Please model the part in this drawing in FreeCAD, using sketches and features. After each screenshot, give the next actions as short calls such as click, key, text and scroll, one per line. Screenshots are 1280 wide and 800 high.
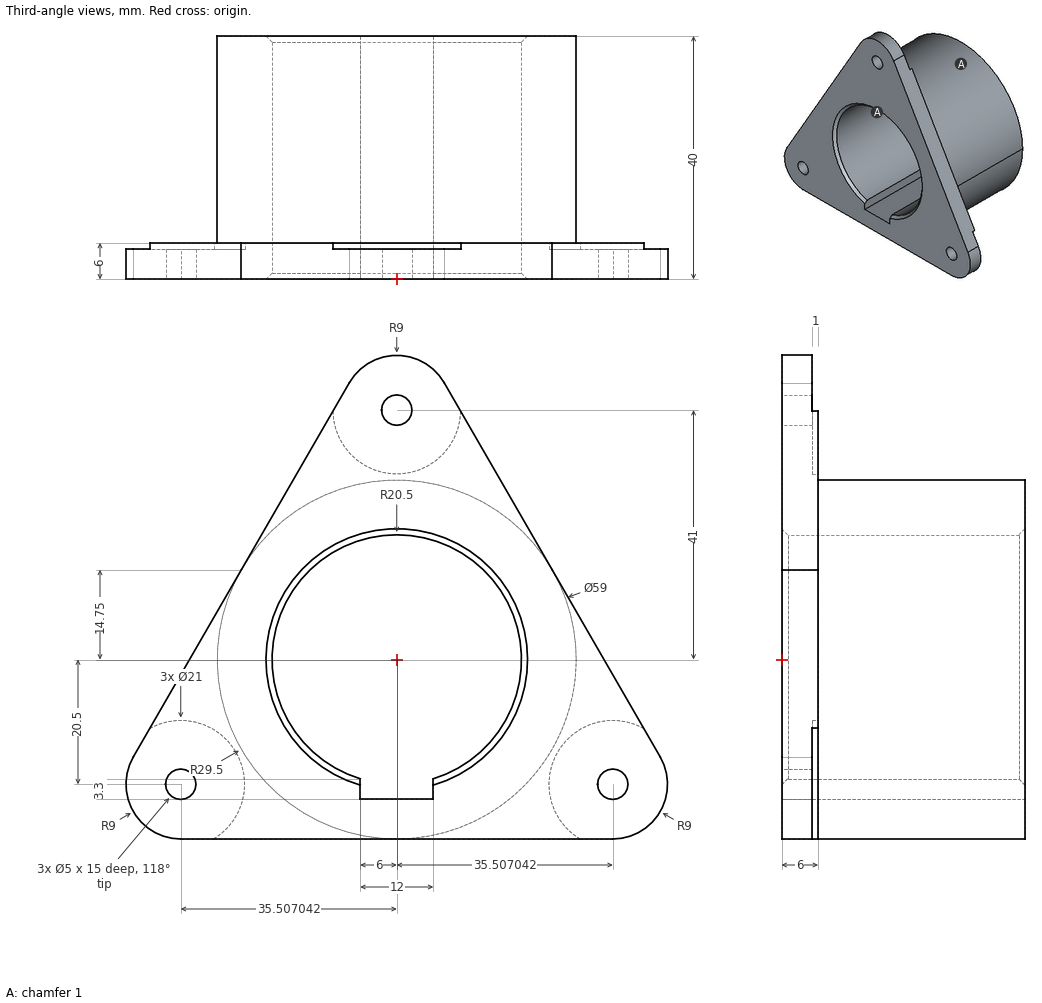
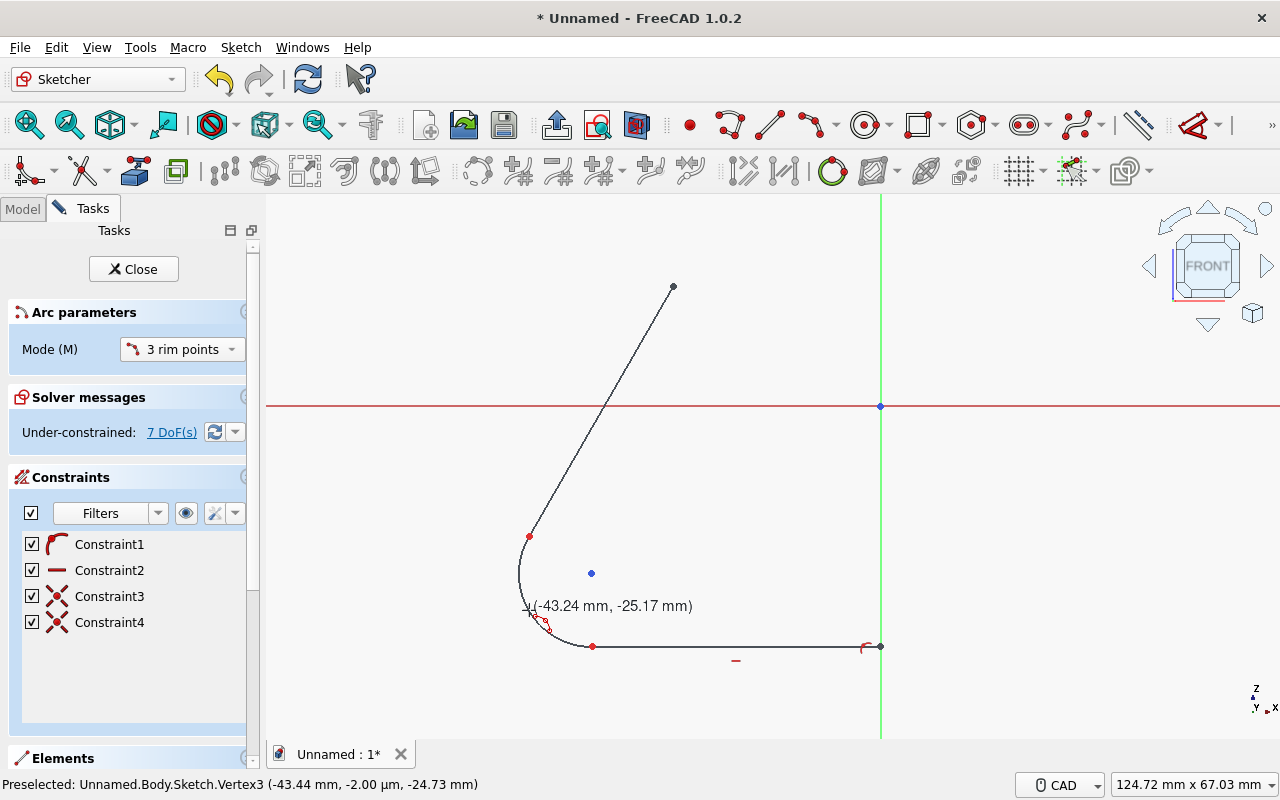
click(673, 287)
click(881, 647)
click(673, 526)
key(Escape)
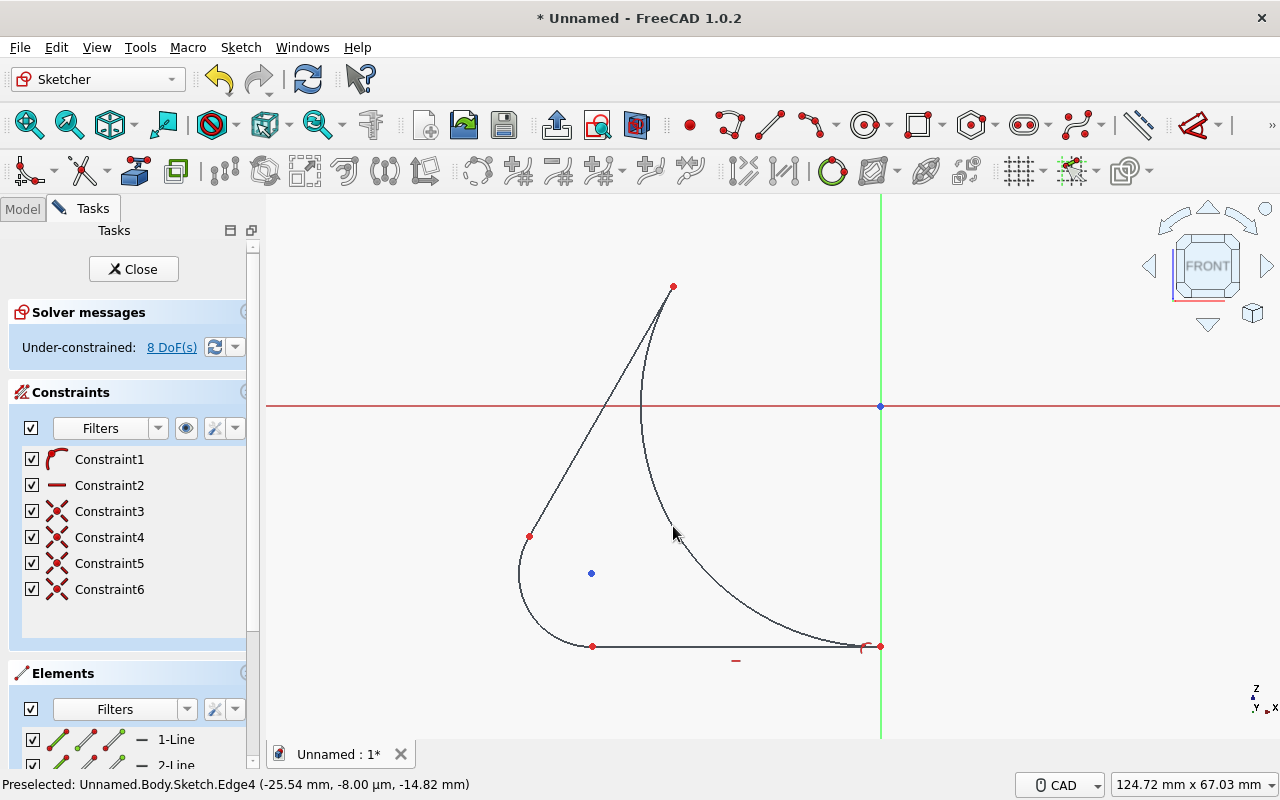
click(794, 647)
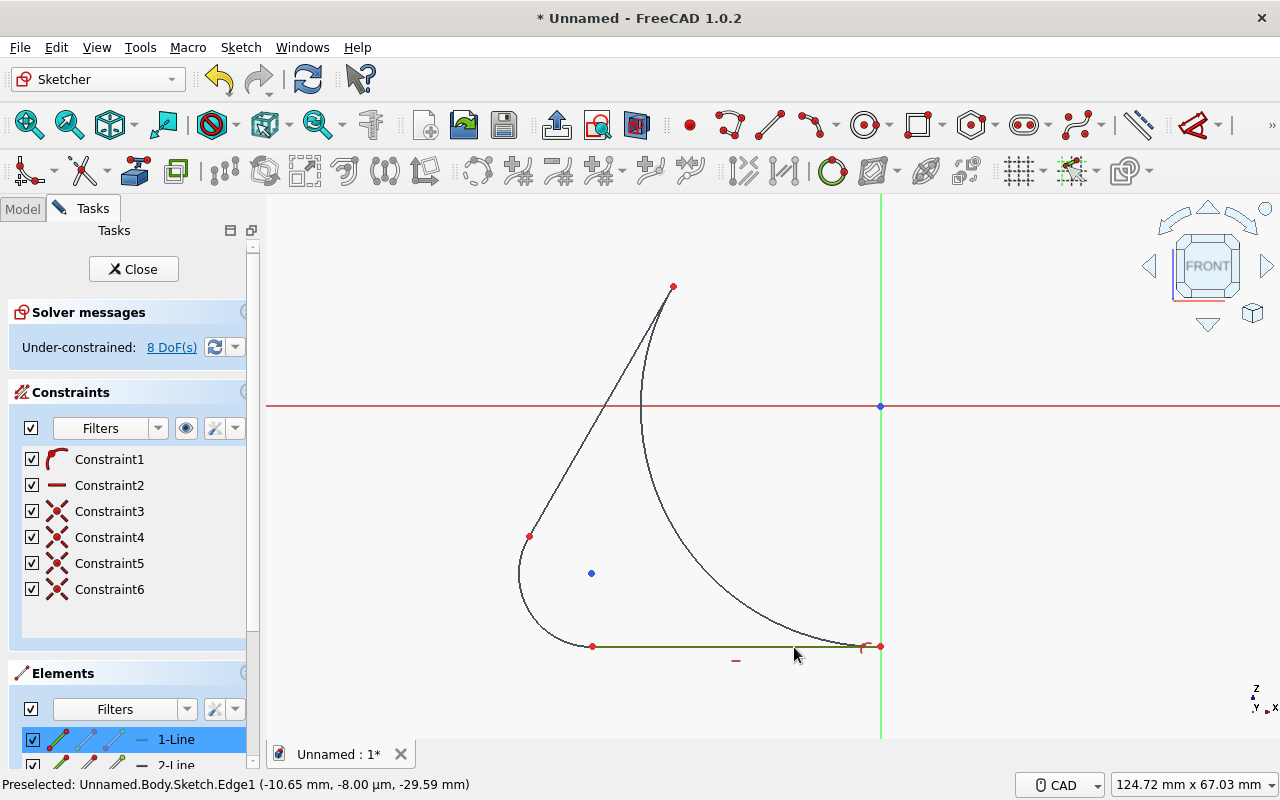
click(519, 581)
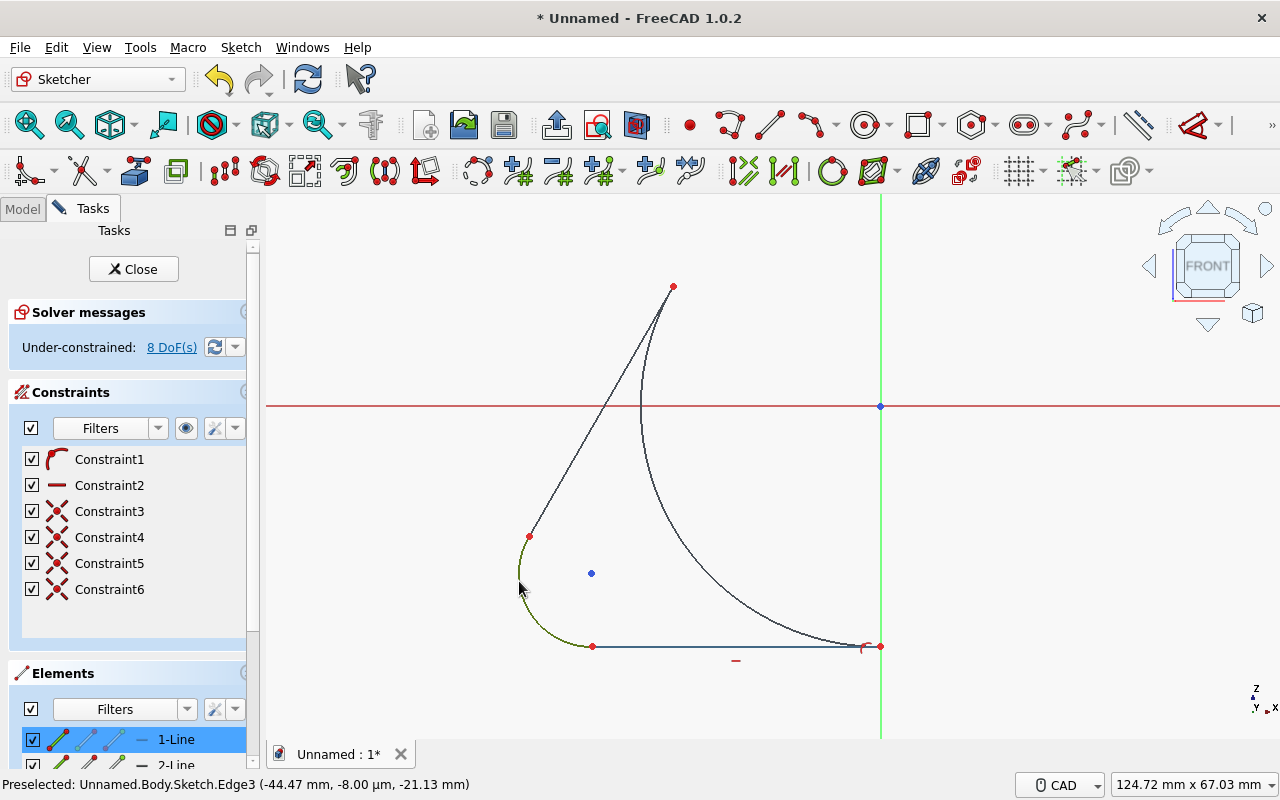
key(t)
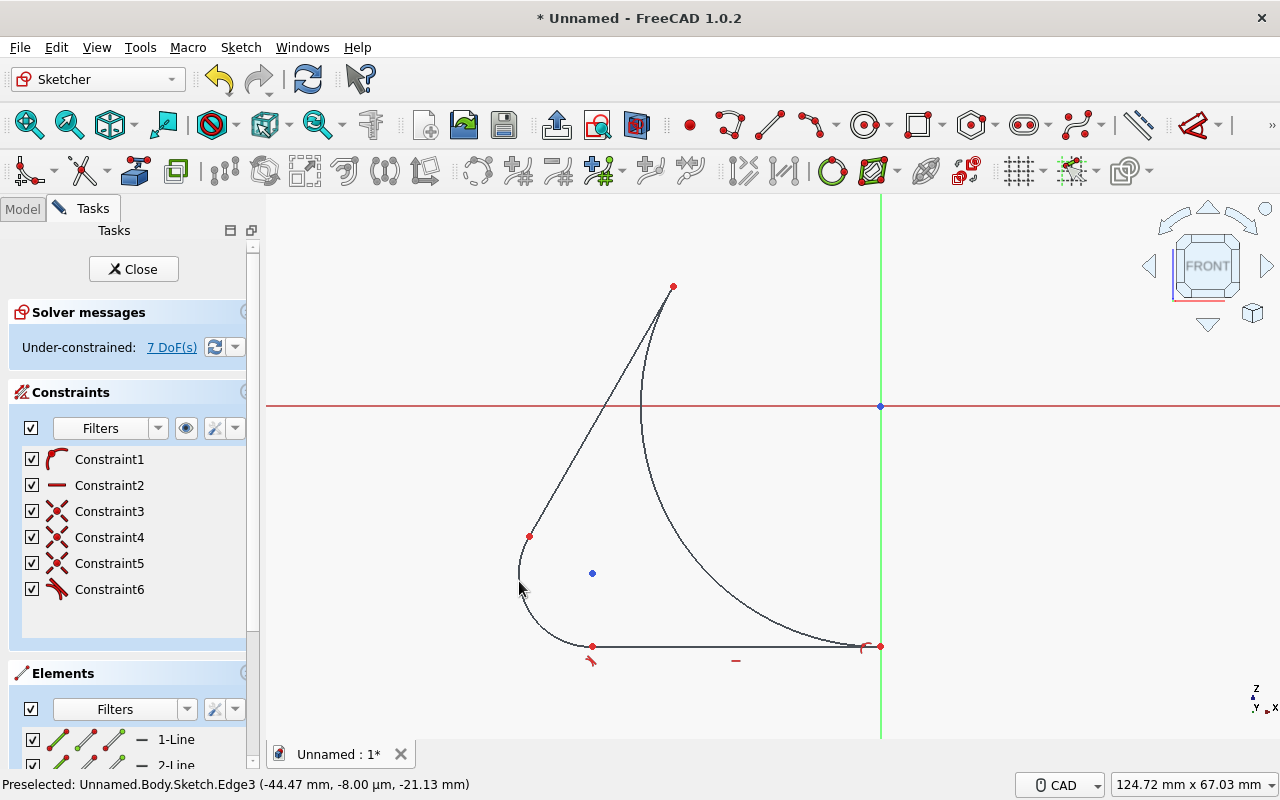
click(794, 647)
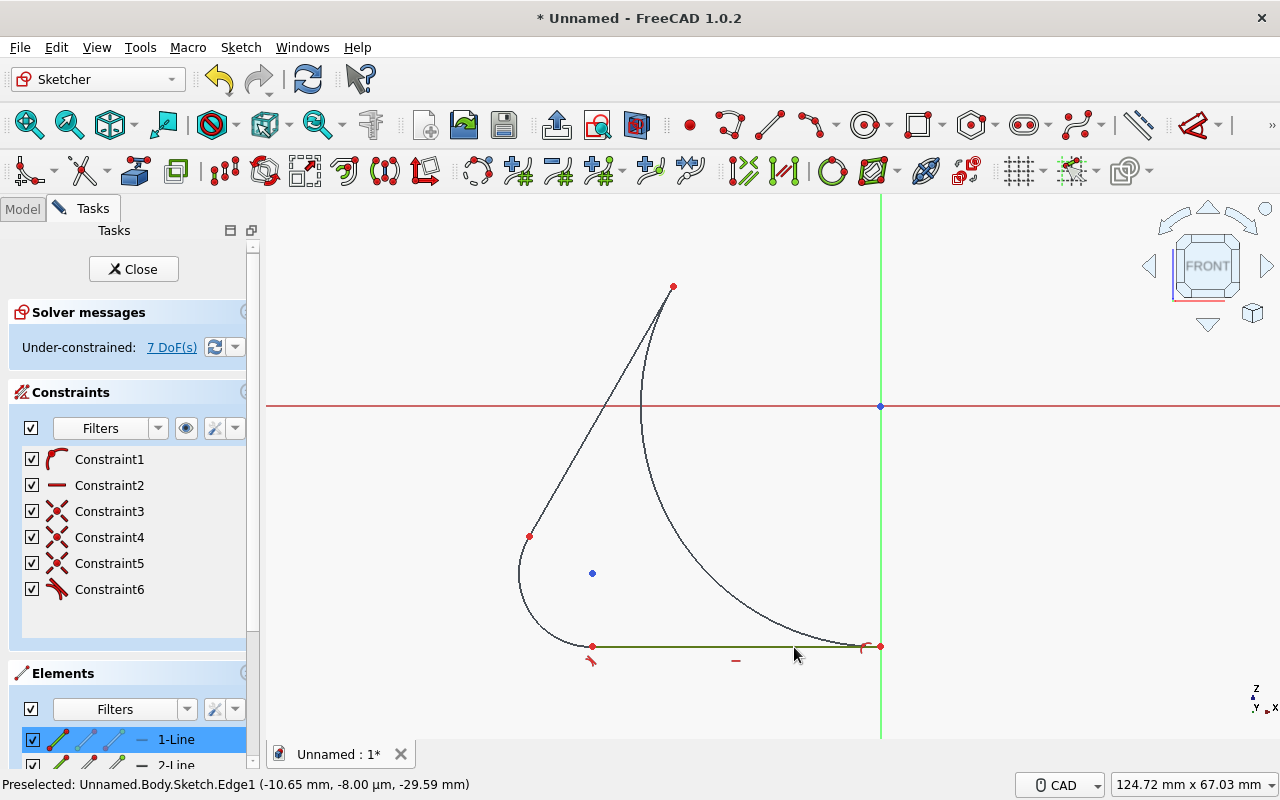
click(642, 432)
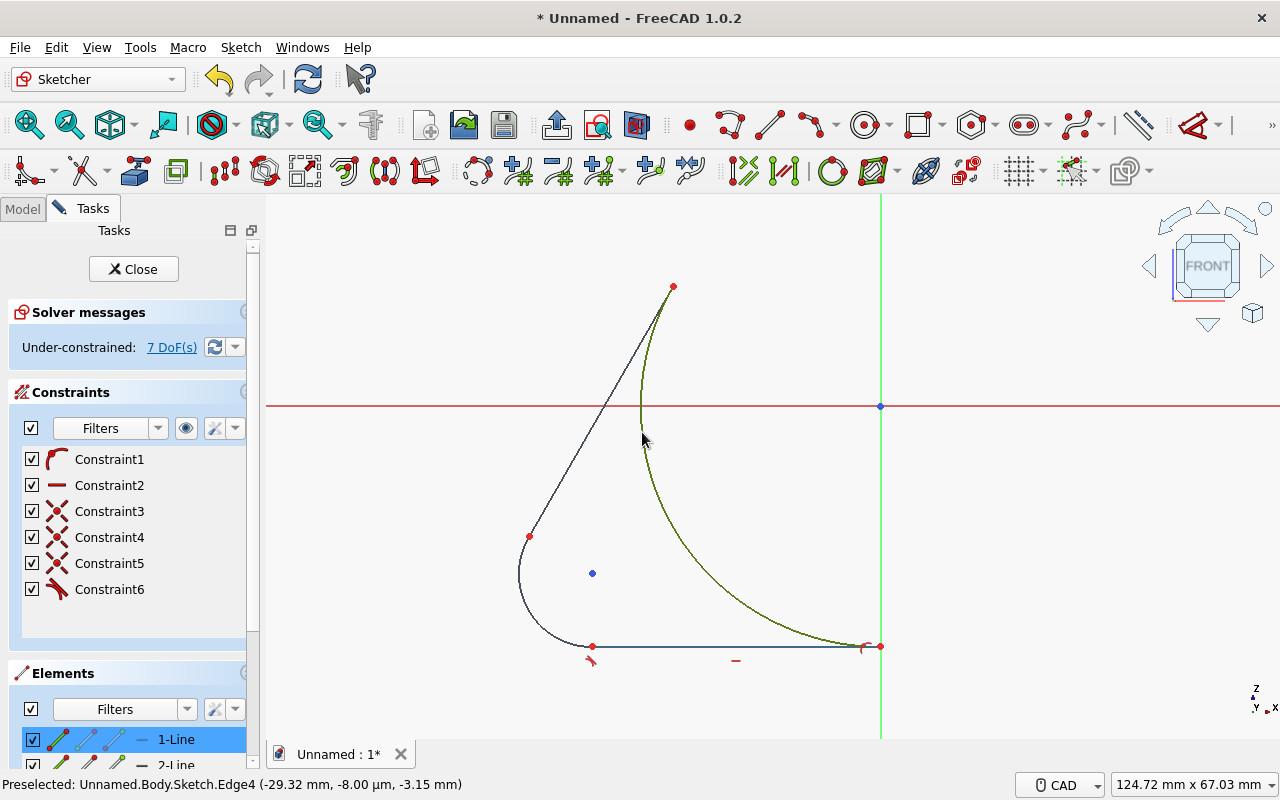
key(t)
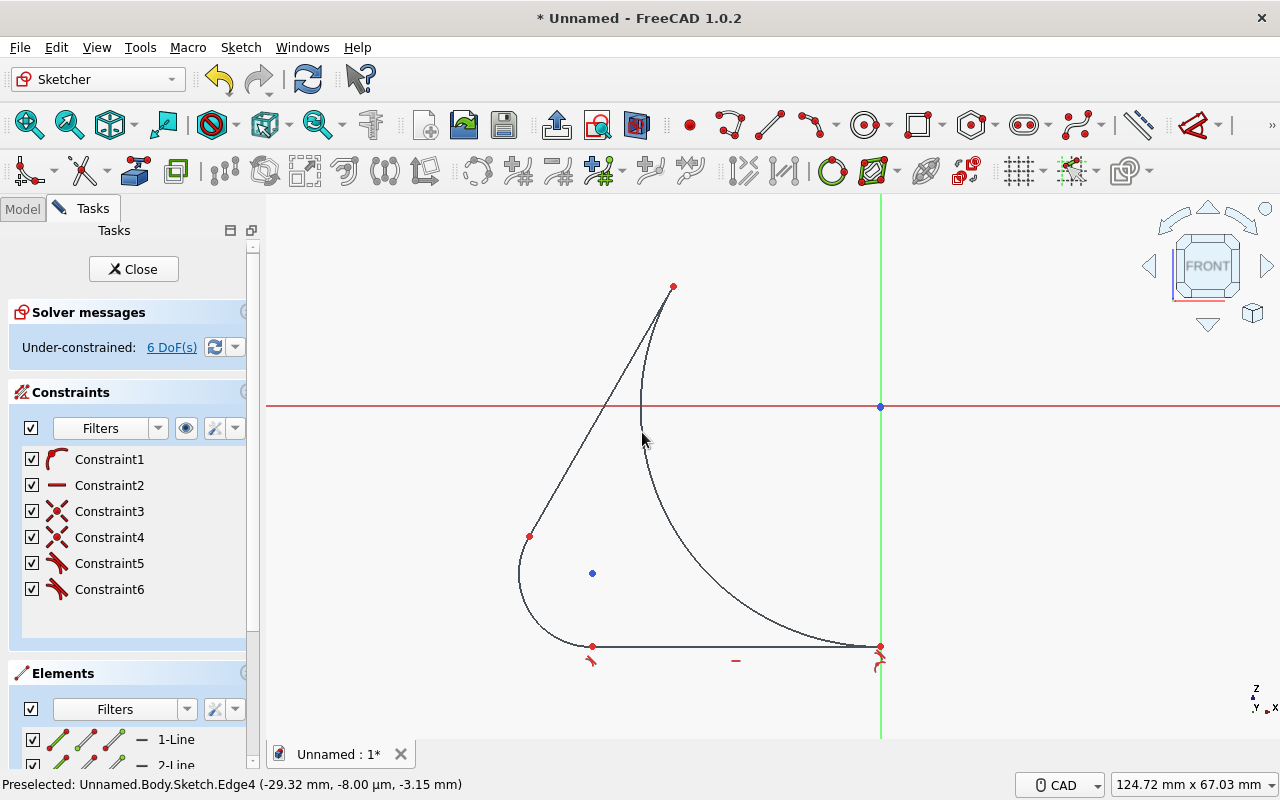
click(572, 462)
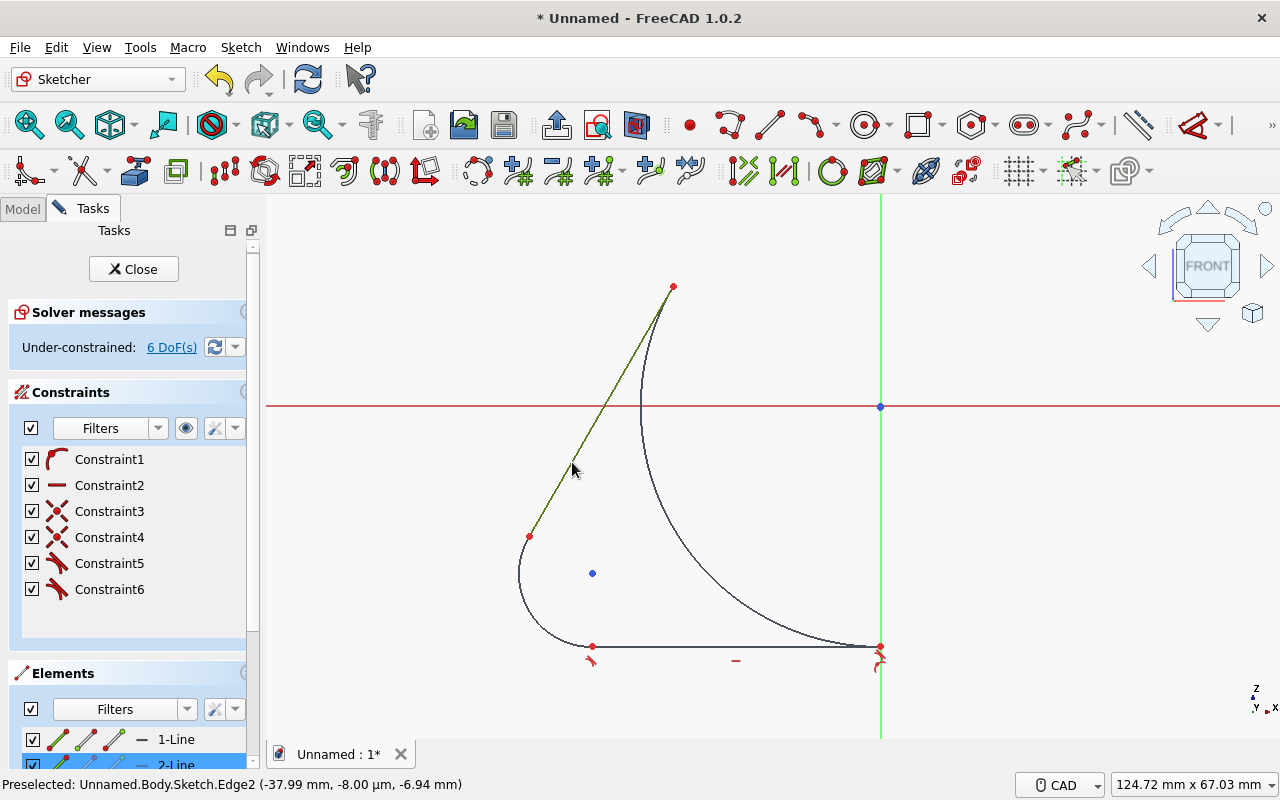
click(519, 581)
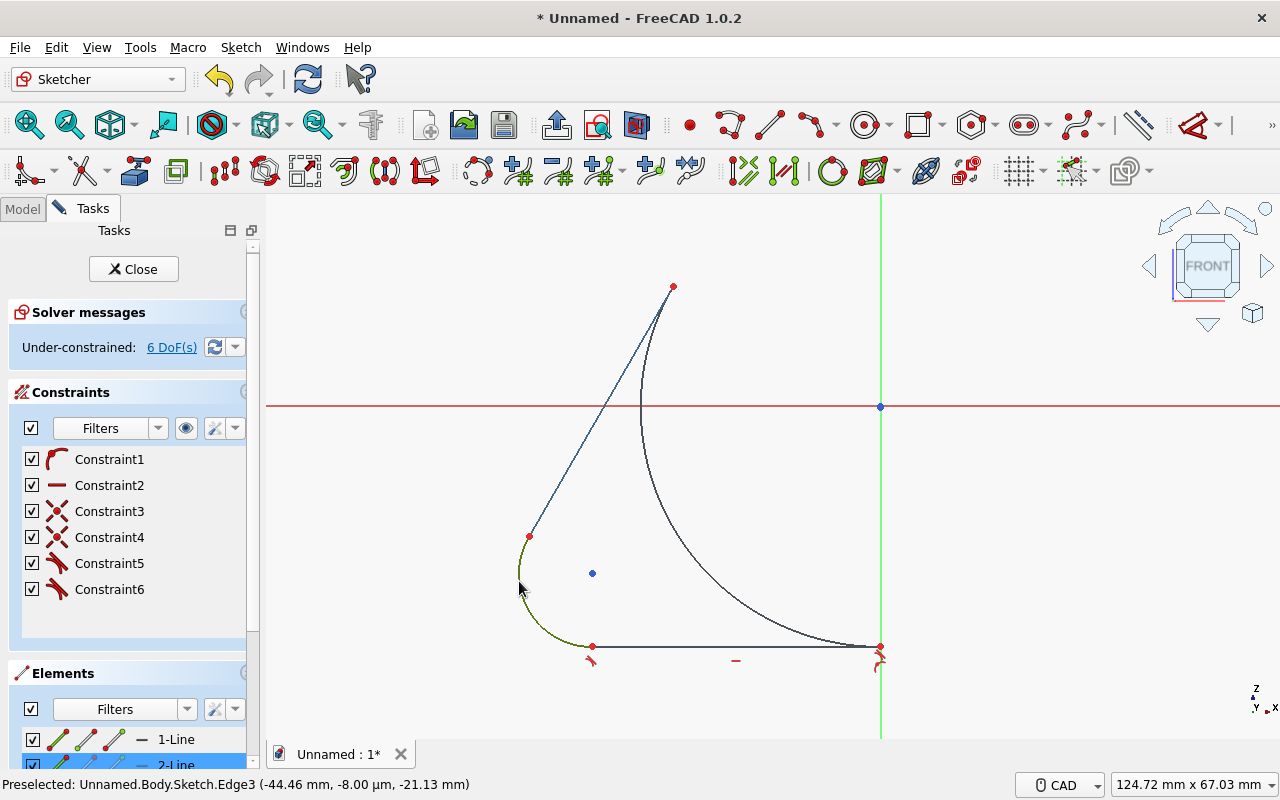
key(t)